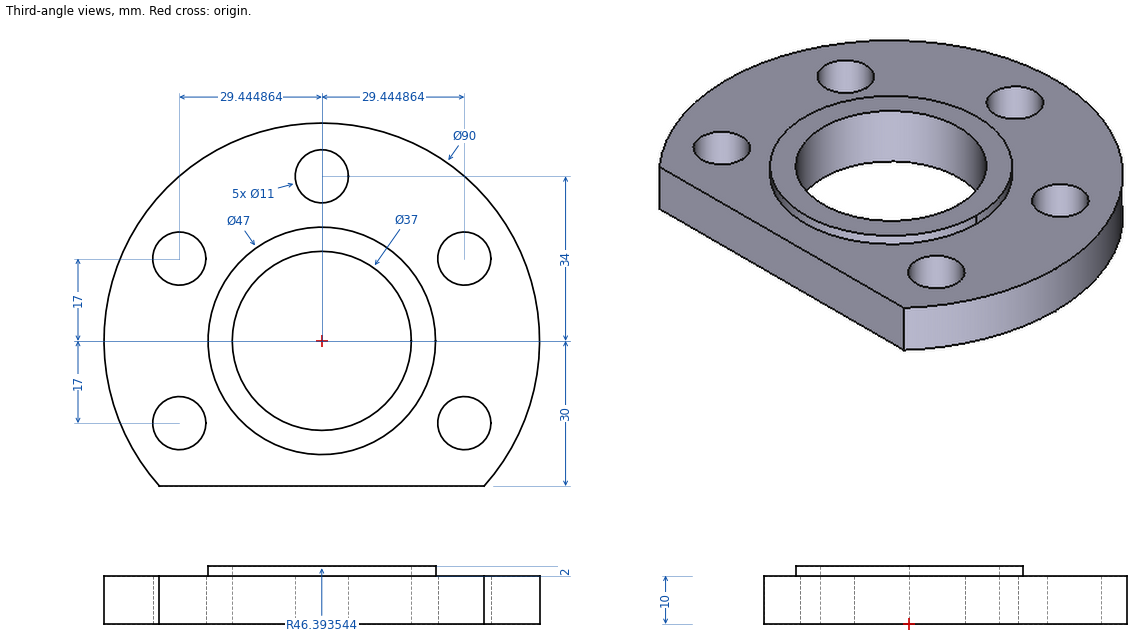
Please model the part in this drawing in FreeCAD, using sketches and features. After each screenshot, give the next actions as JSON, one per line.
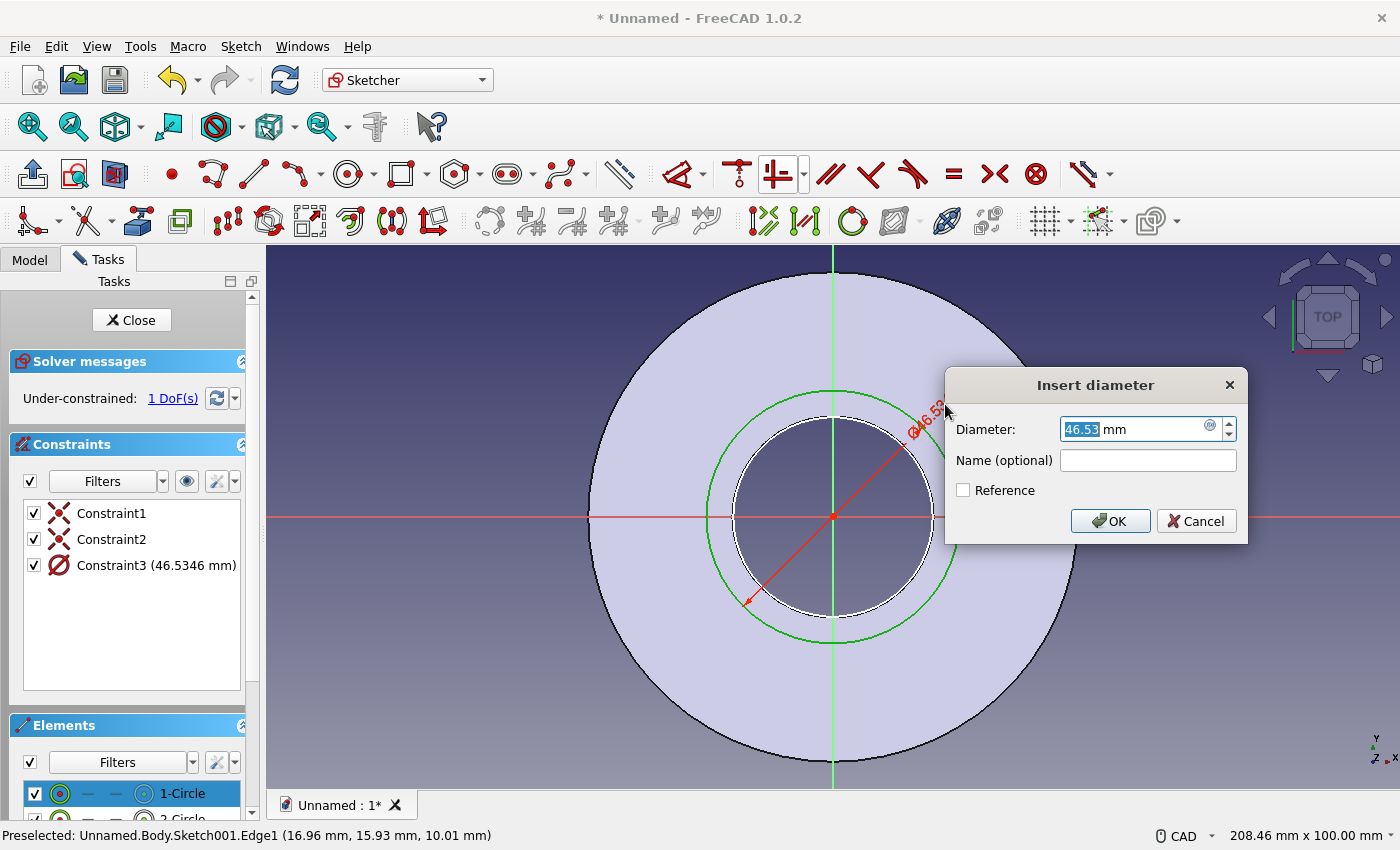
{"action": "type", "text": "47"}
{"action": "key", "text": "Return"}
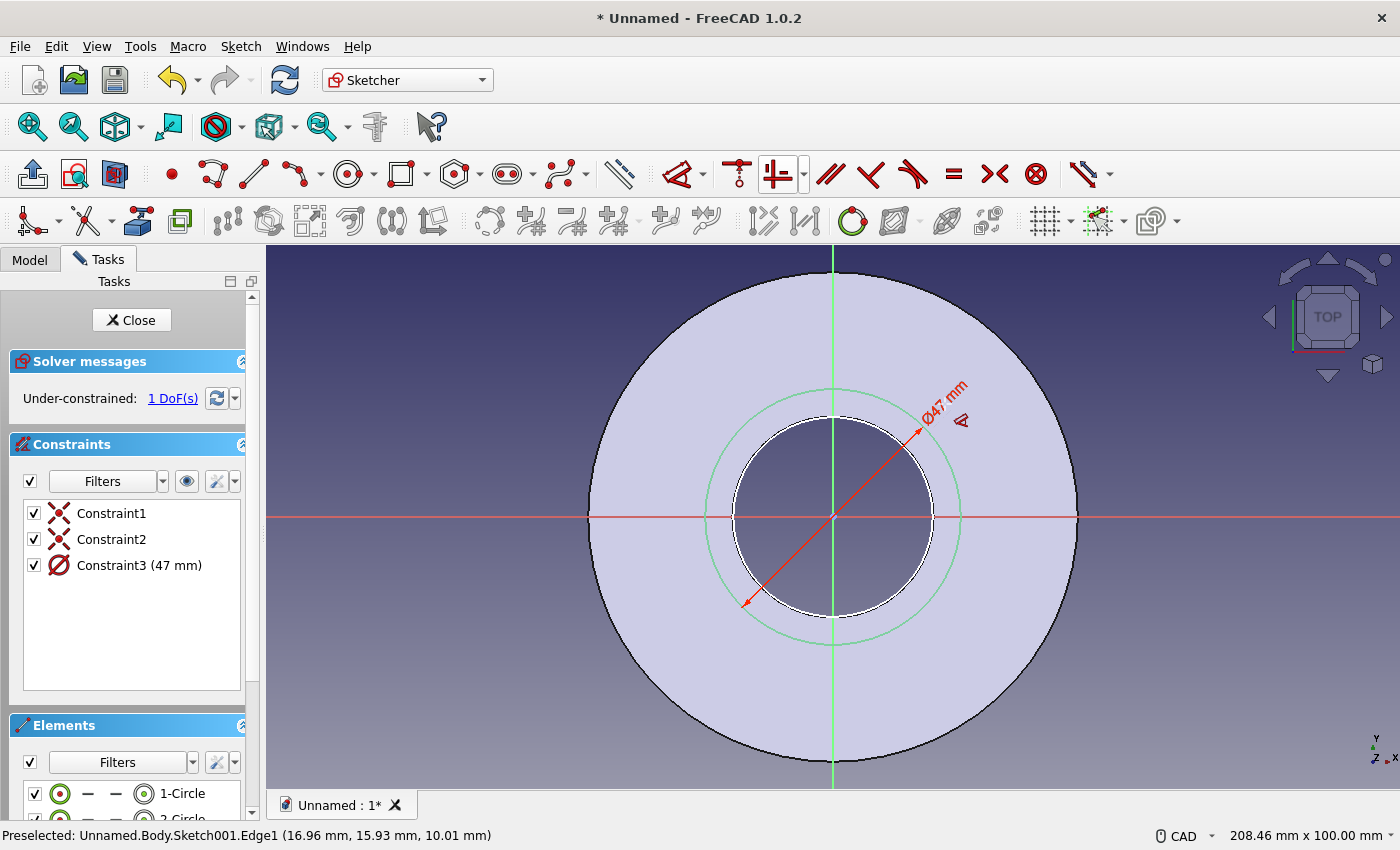
{"action": "left_click", "coordinate": [903, 446]}
{"action": "left_click", "coordinate": [981, 472]}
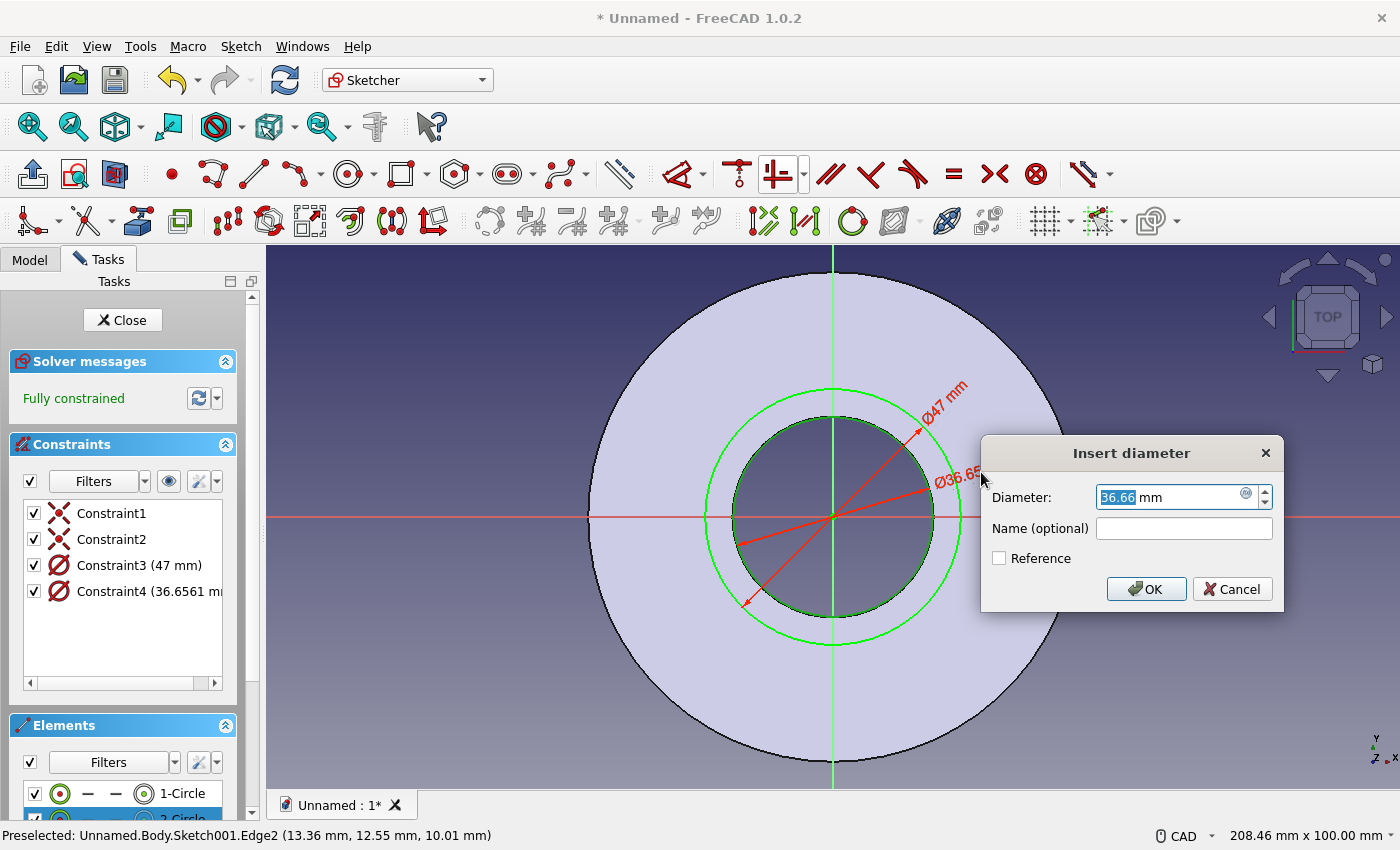
{"action": "type", "text": "37"}
{"action": "key", "text": "Return"}
{"action": "key", "text": "Escape"}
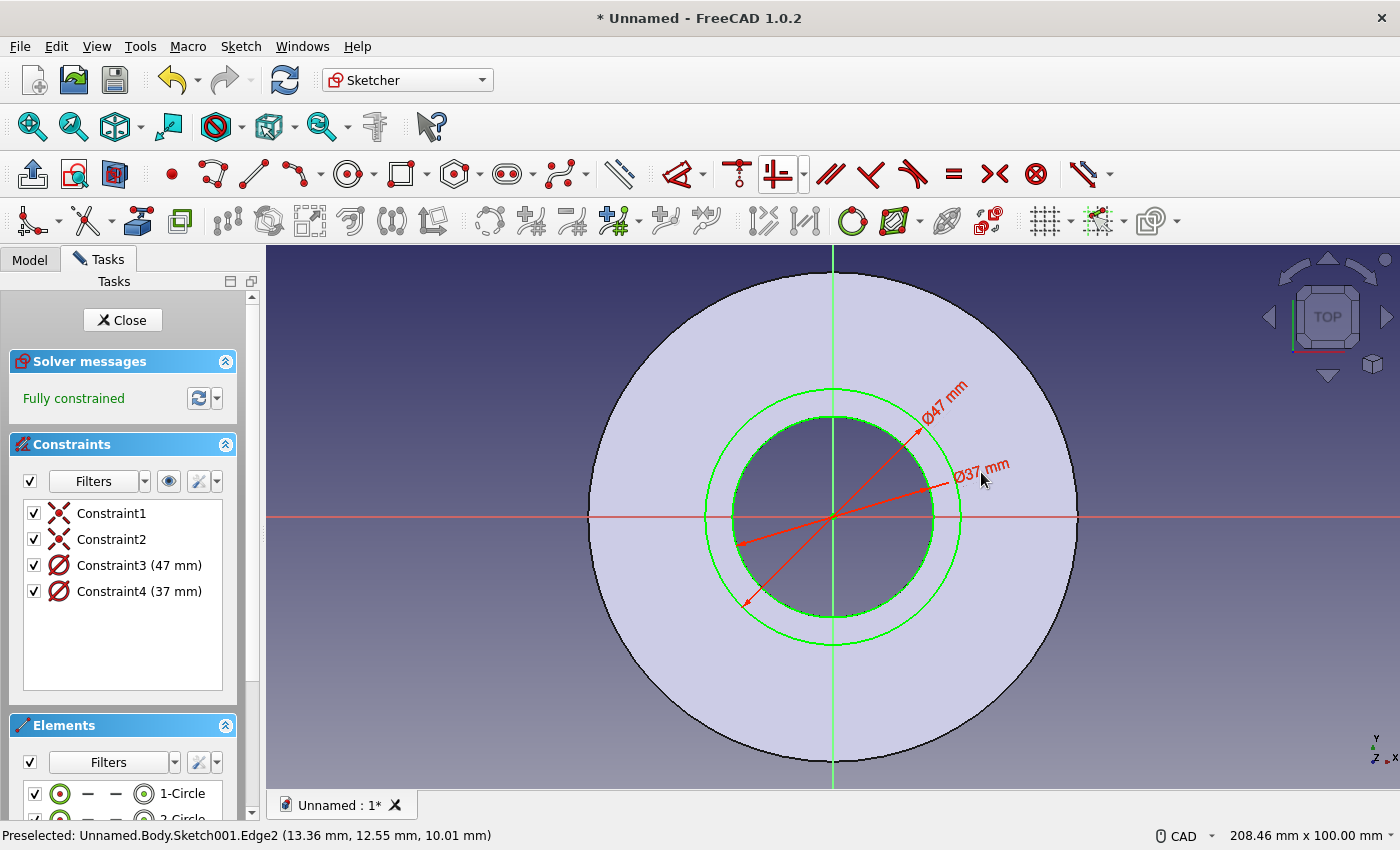
{"action": "left_click", "coordinate": [123, 320]}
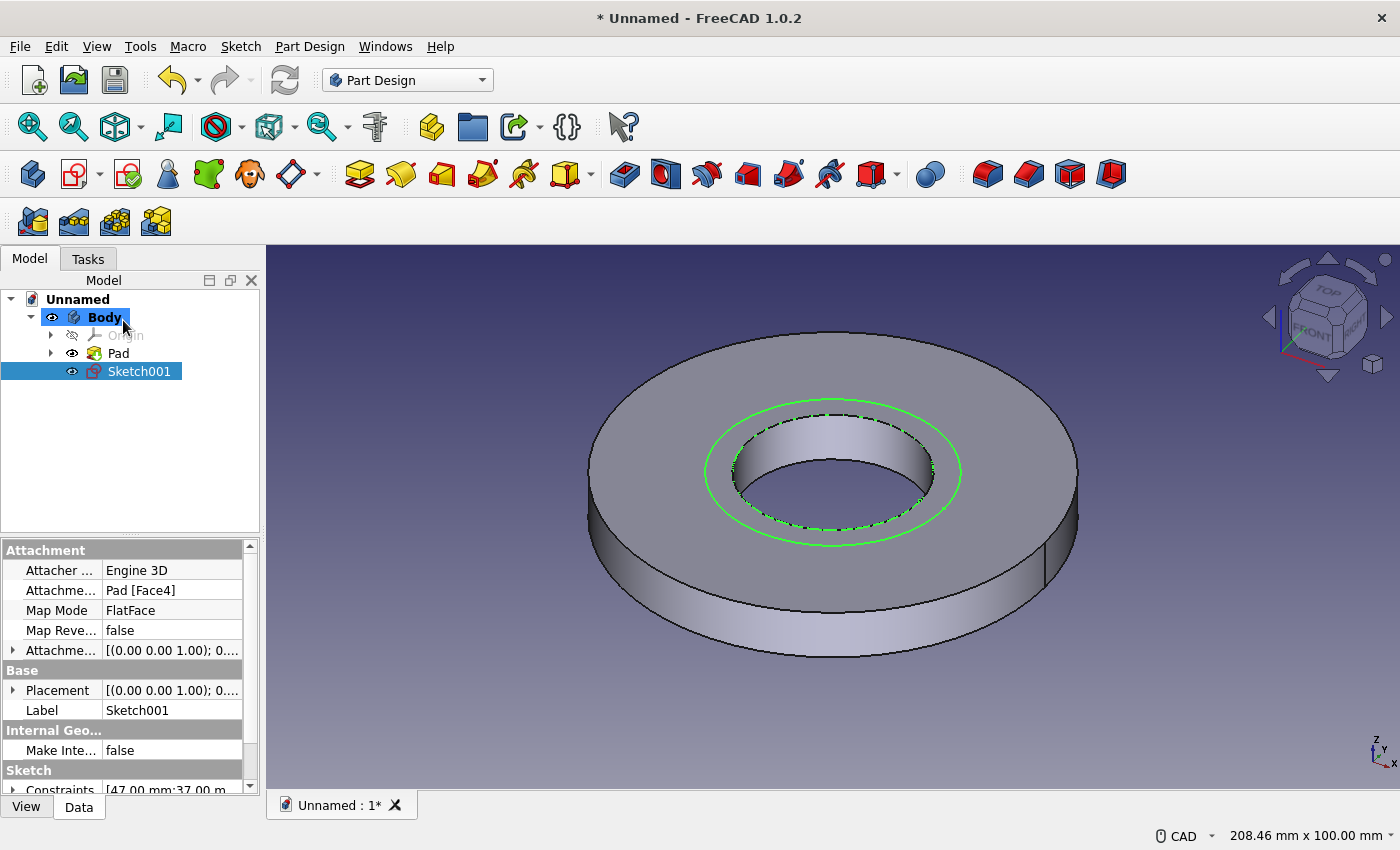
{"action": "left_click", "coordinate": [360, 174]}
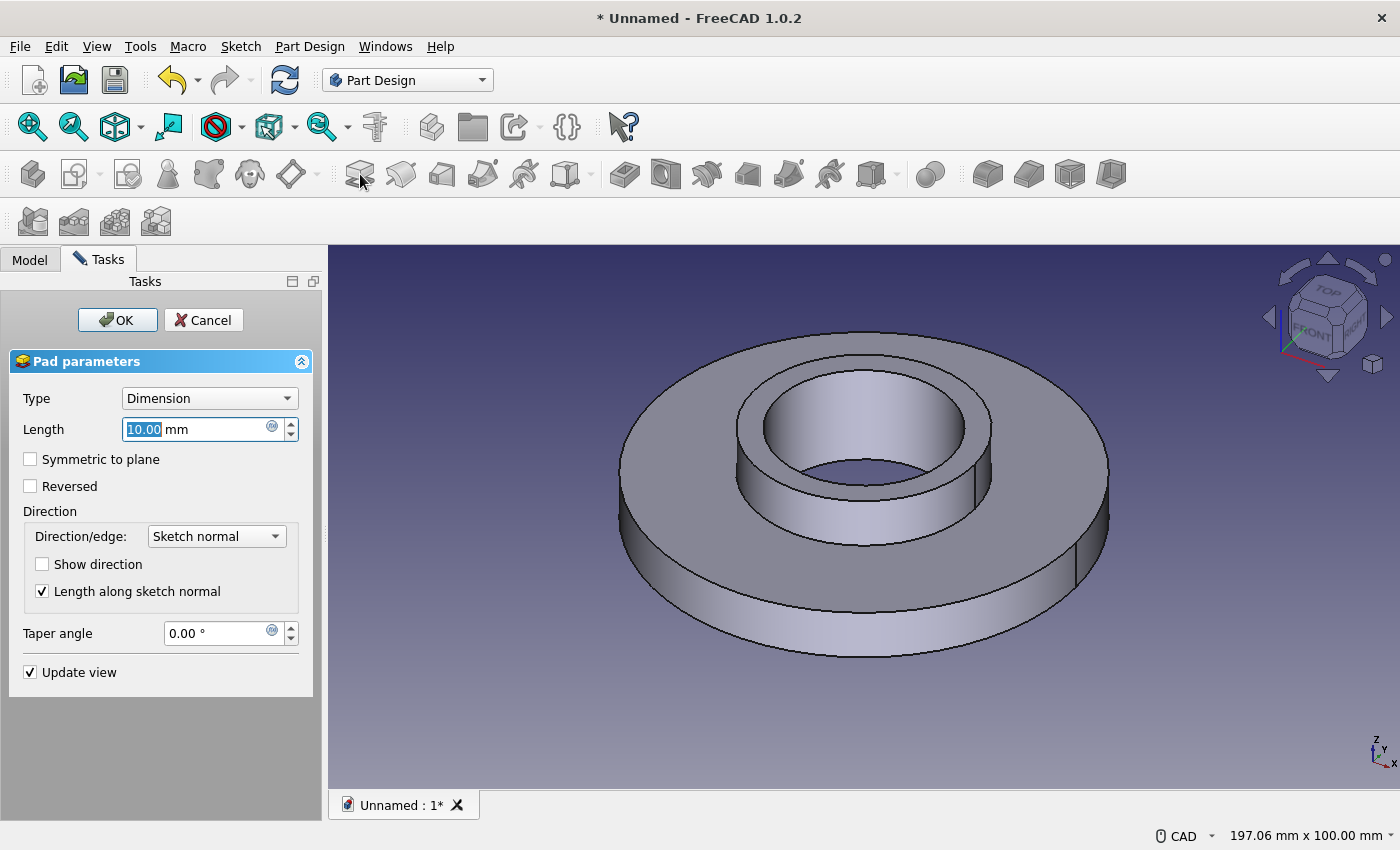
{"action": "type", "text": "2"}
{"action": "key", "text": "Tab"}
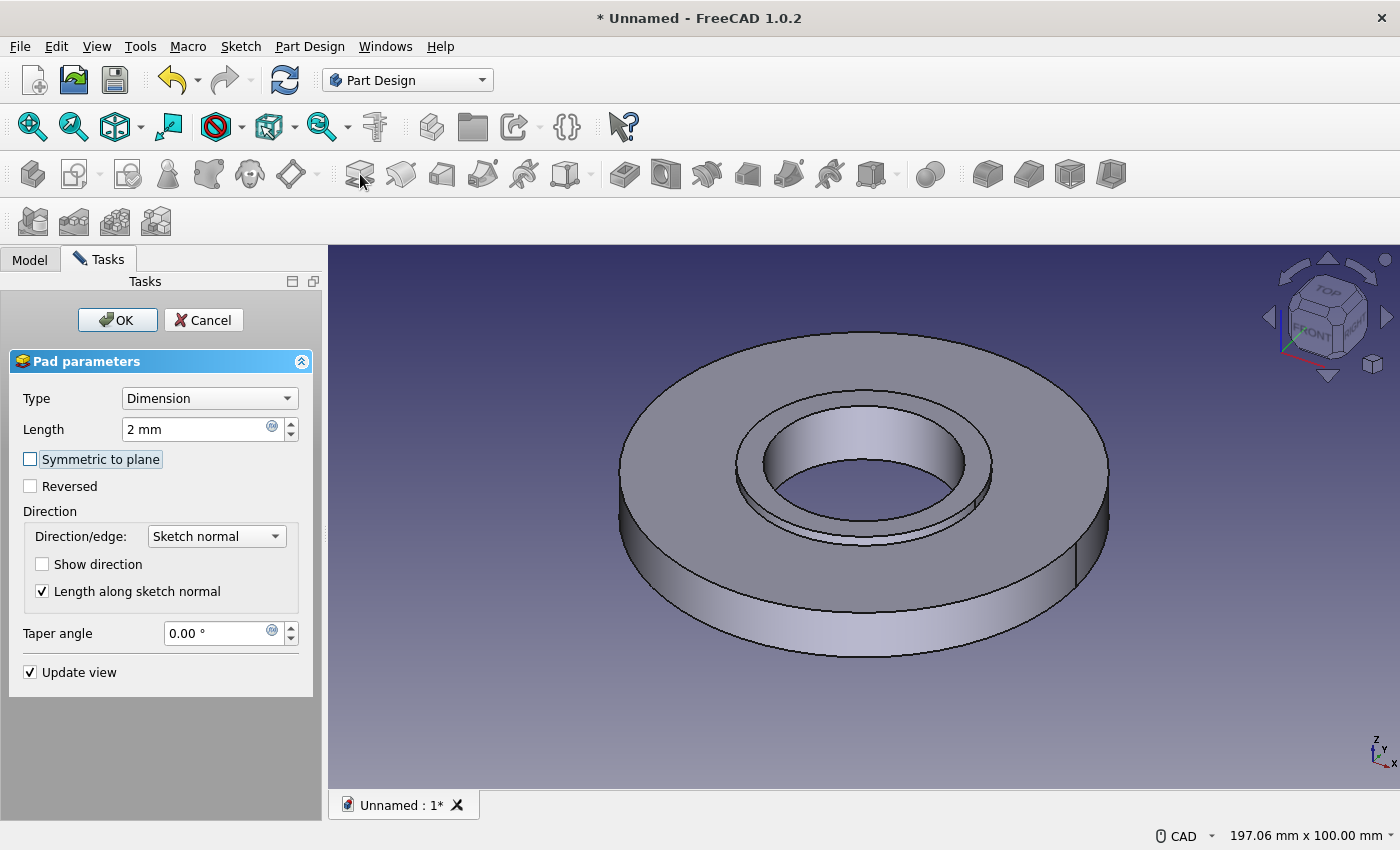
{"action": "left_click", "coordinate": [118, 320]}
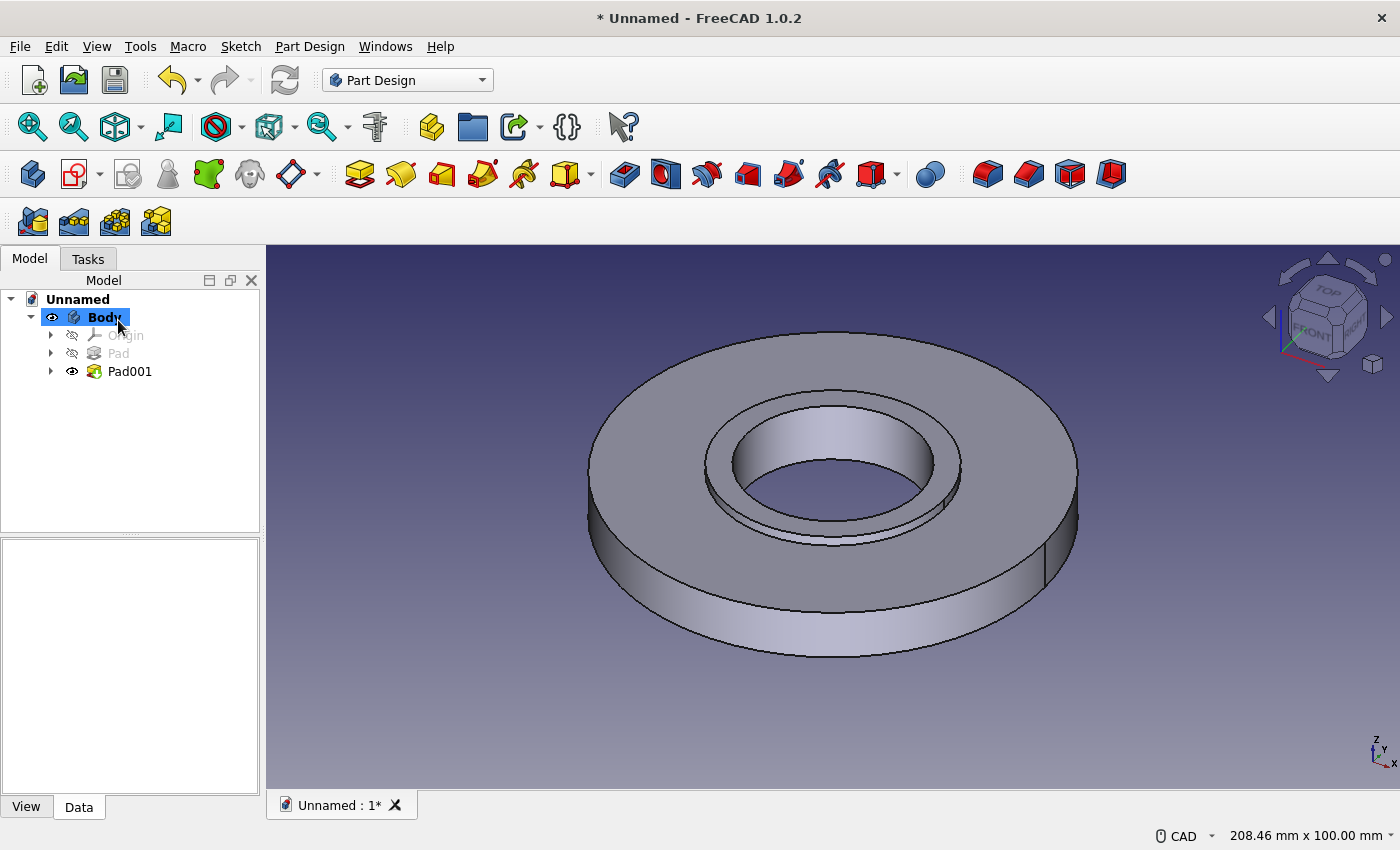
{"action": "left_click", "coordinate": [1024, 442]}